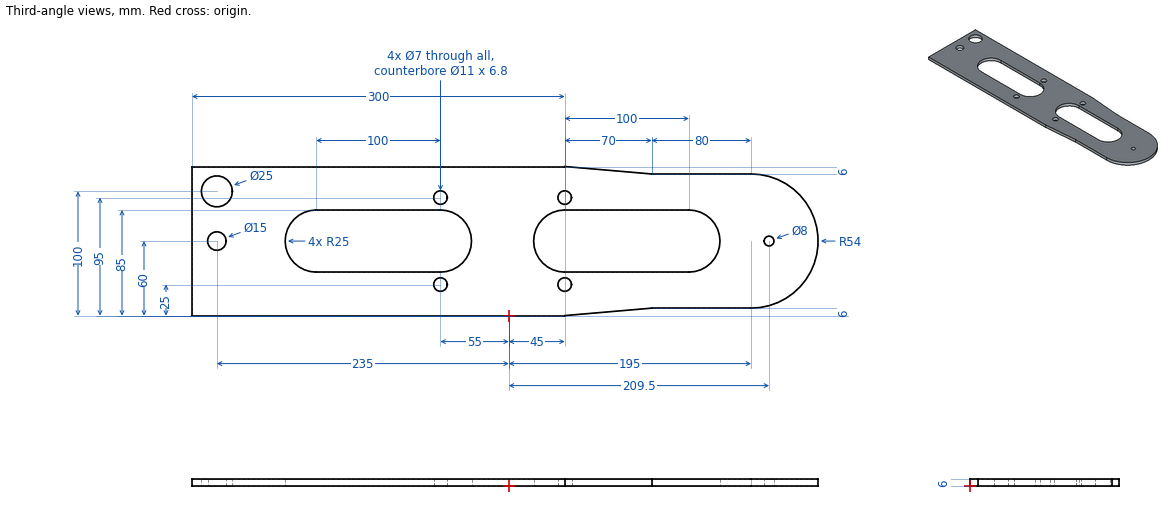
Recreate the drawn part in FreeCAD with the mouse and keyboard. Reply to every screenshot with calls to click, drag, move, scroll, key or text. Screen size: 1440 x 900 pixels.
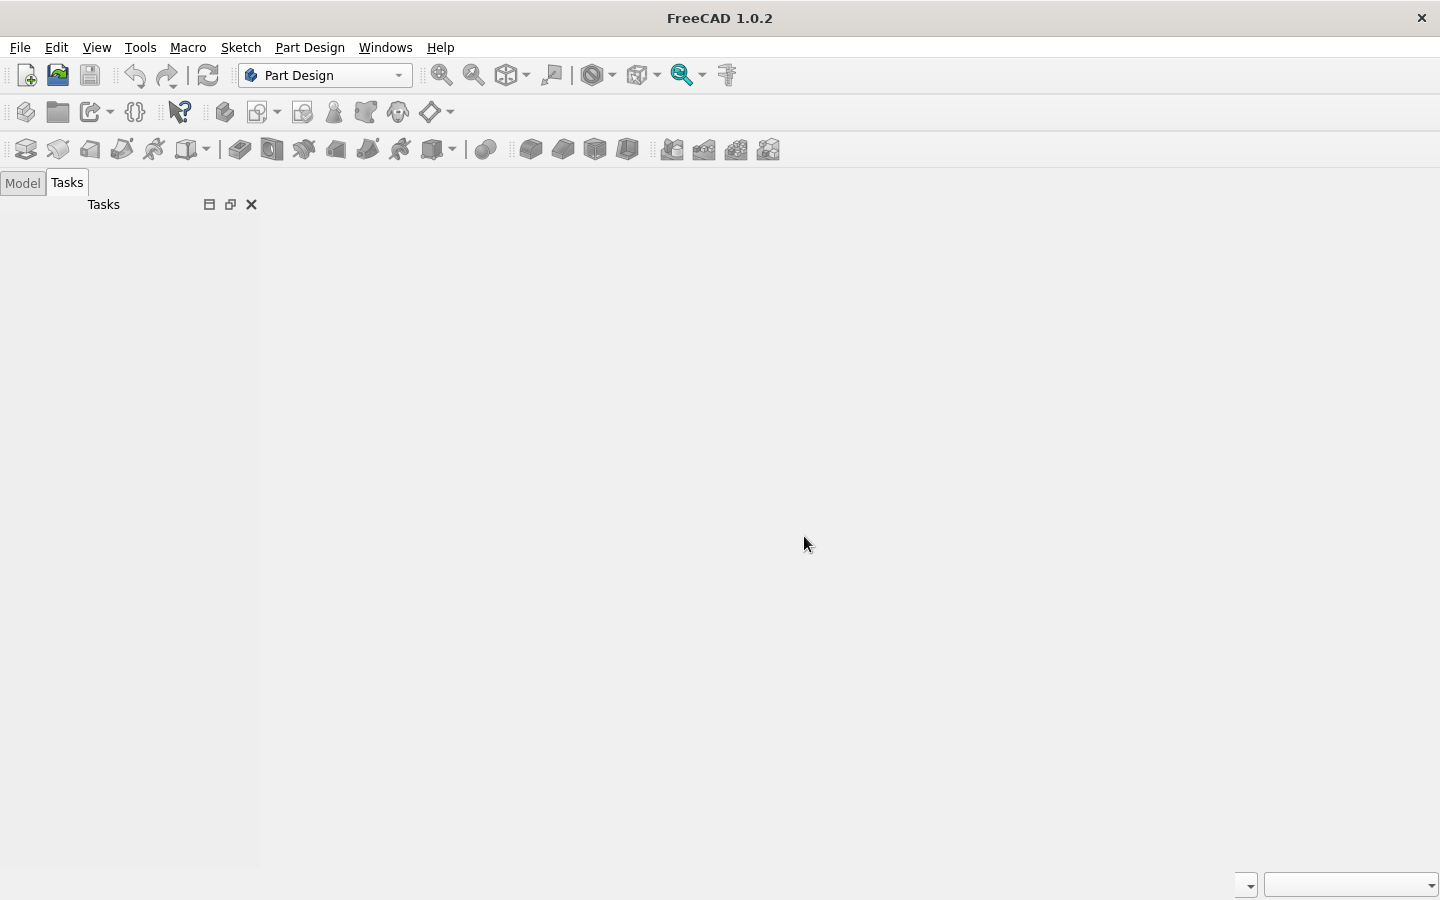
key(ctrl+n)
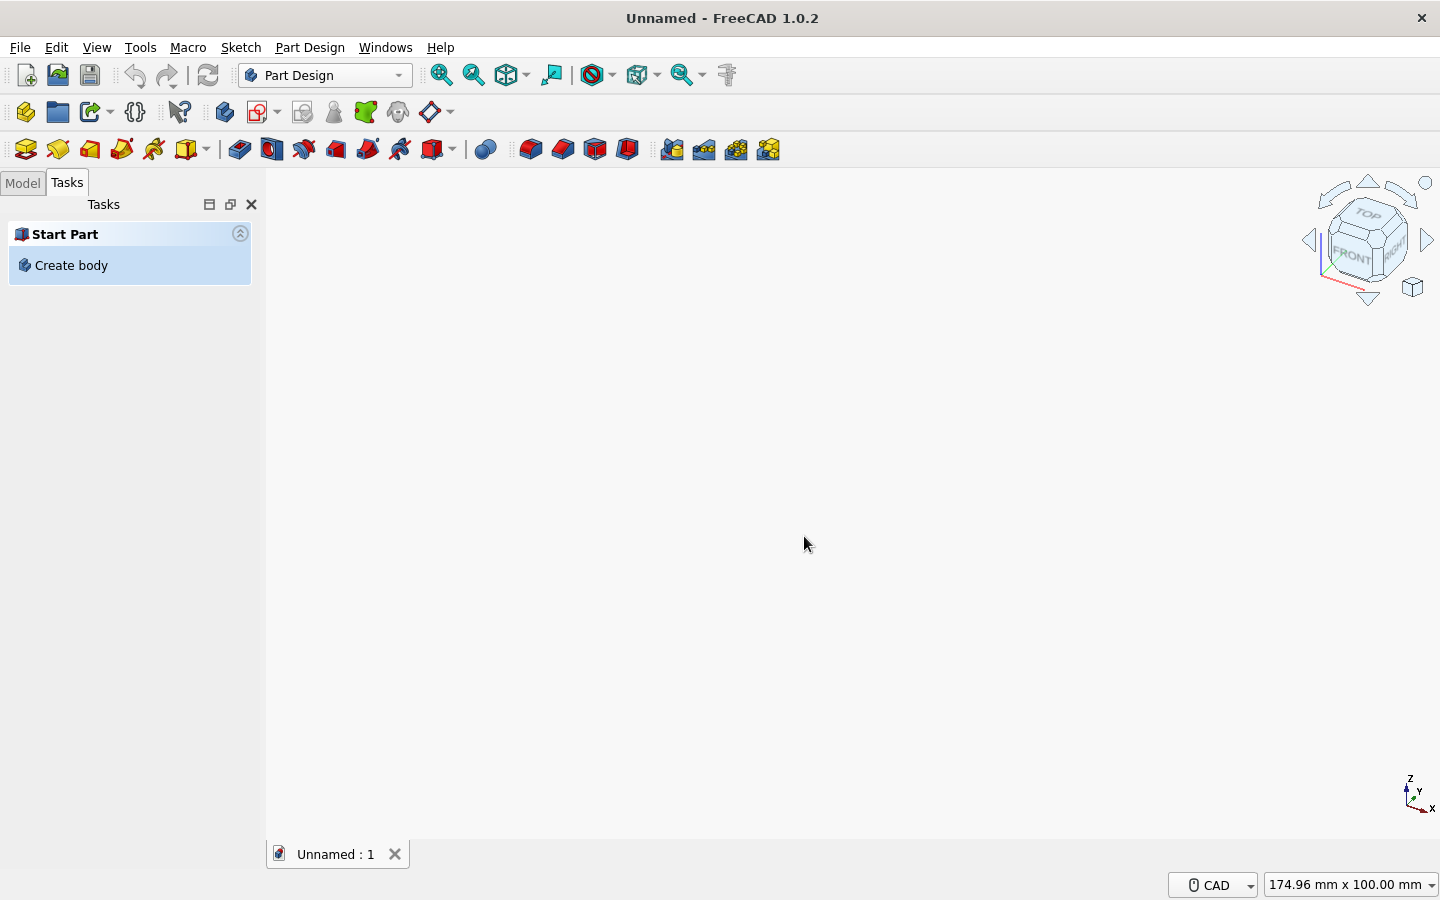
click(258, 112)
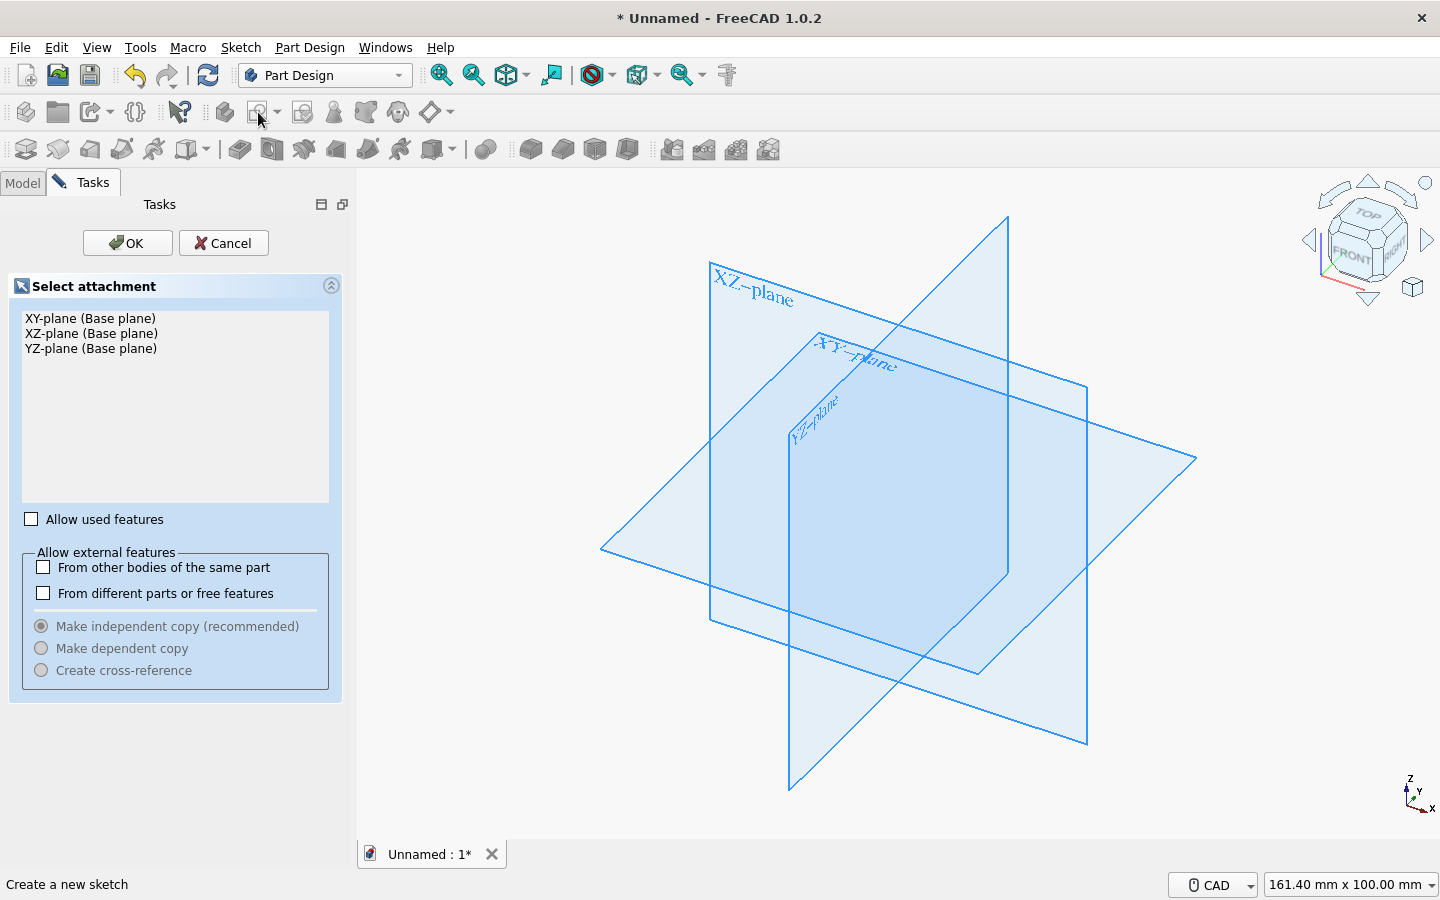
click(82, 318)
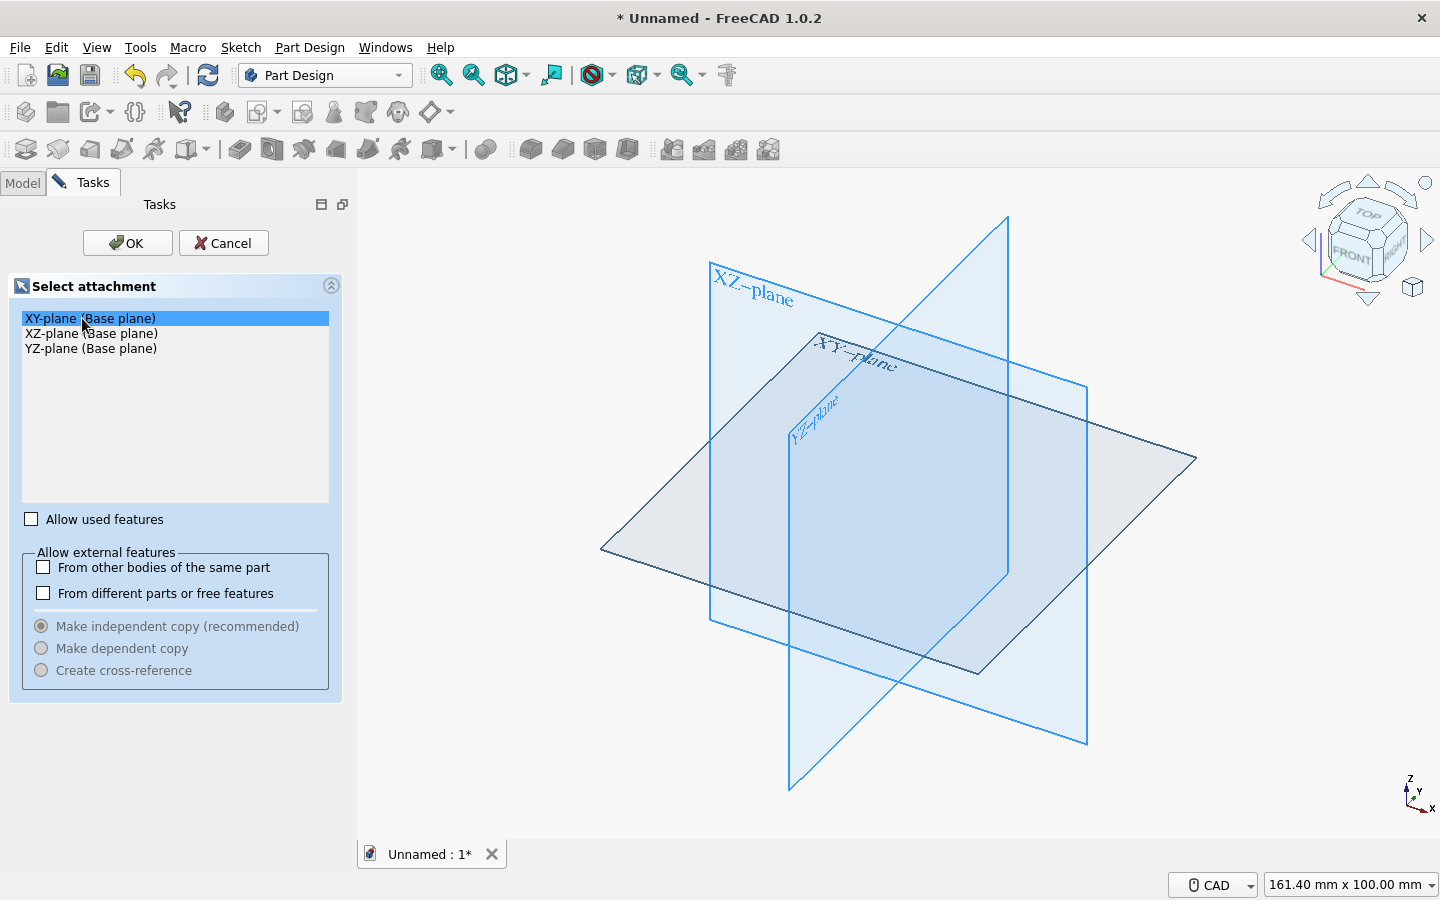
click(128, 243)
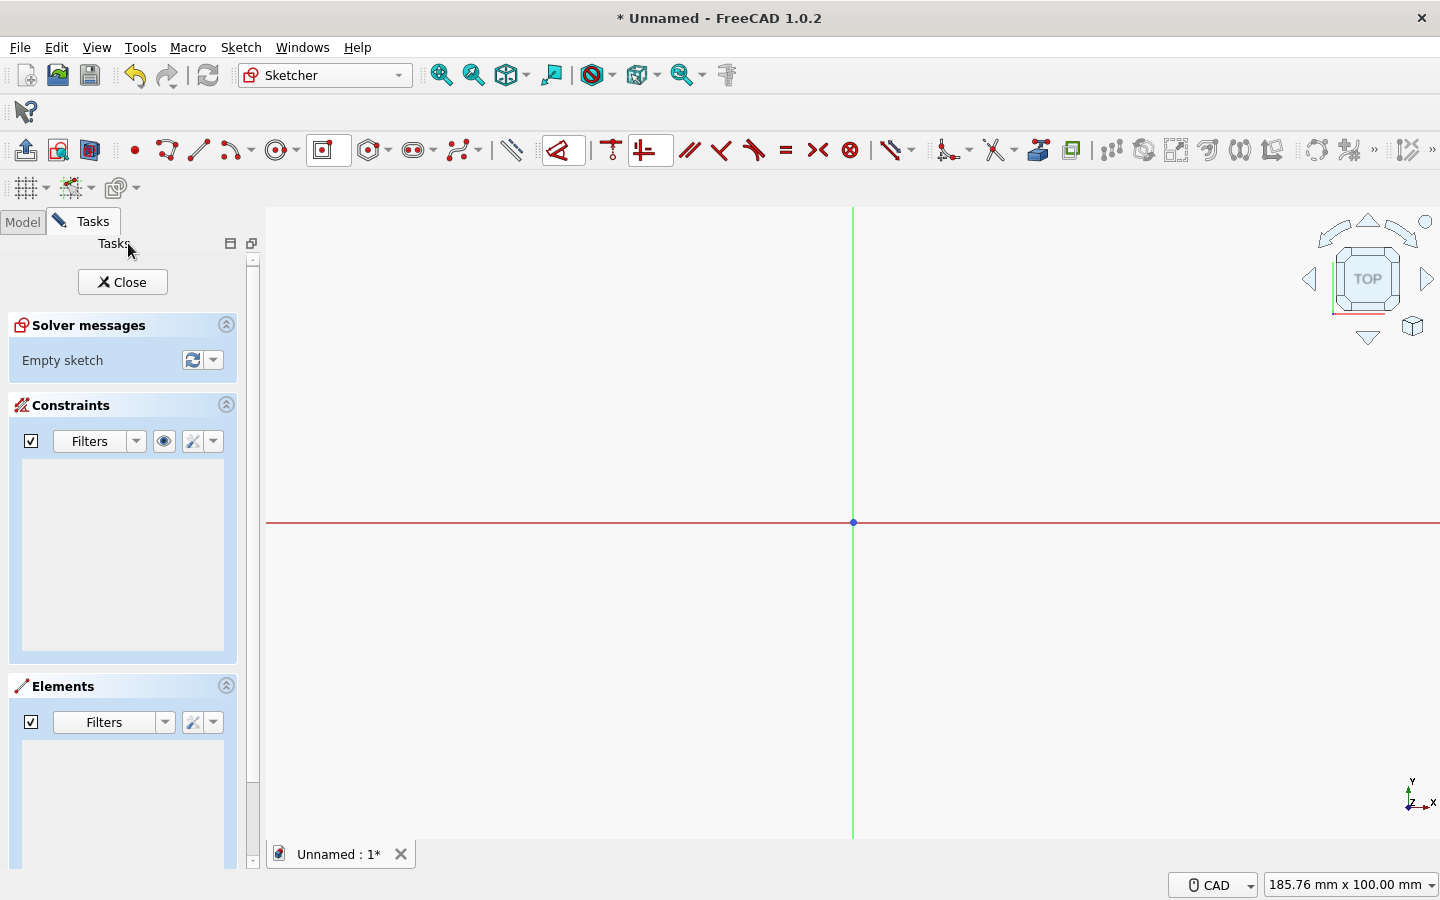
scroll(772, 619, down, 8)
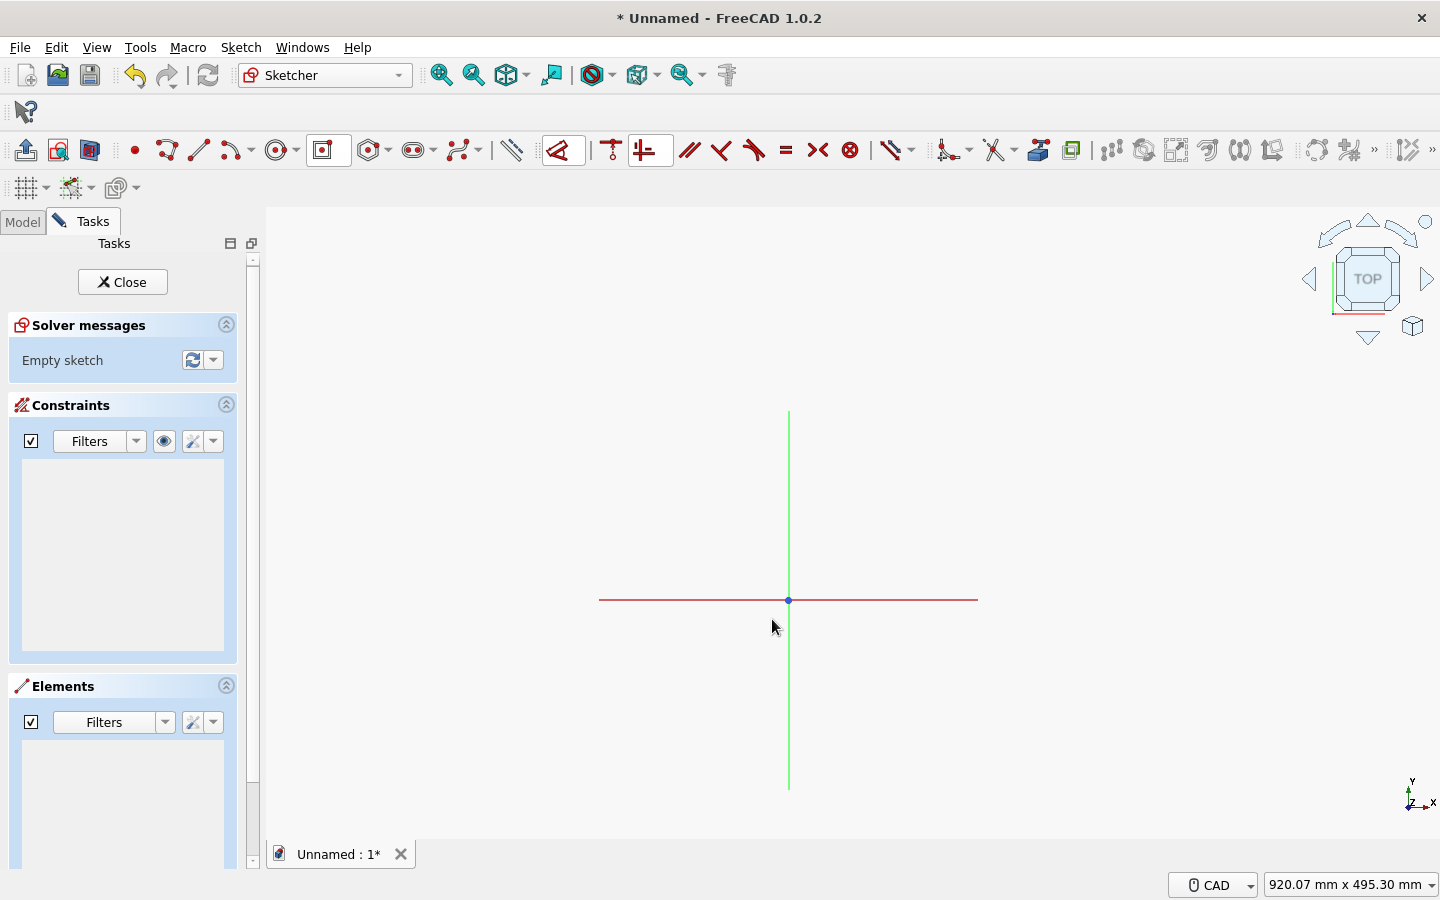
click(168, 150)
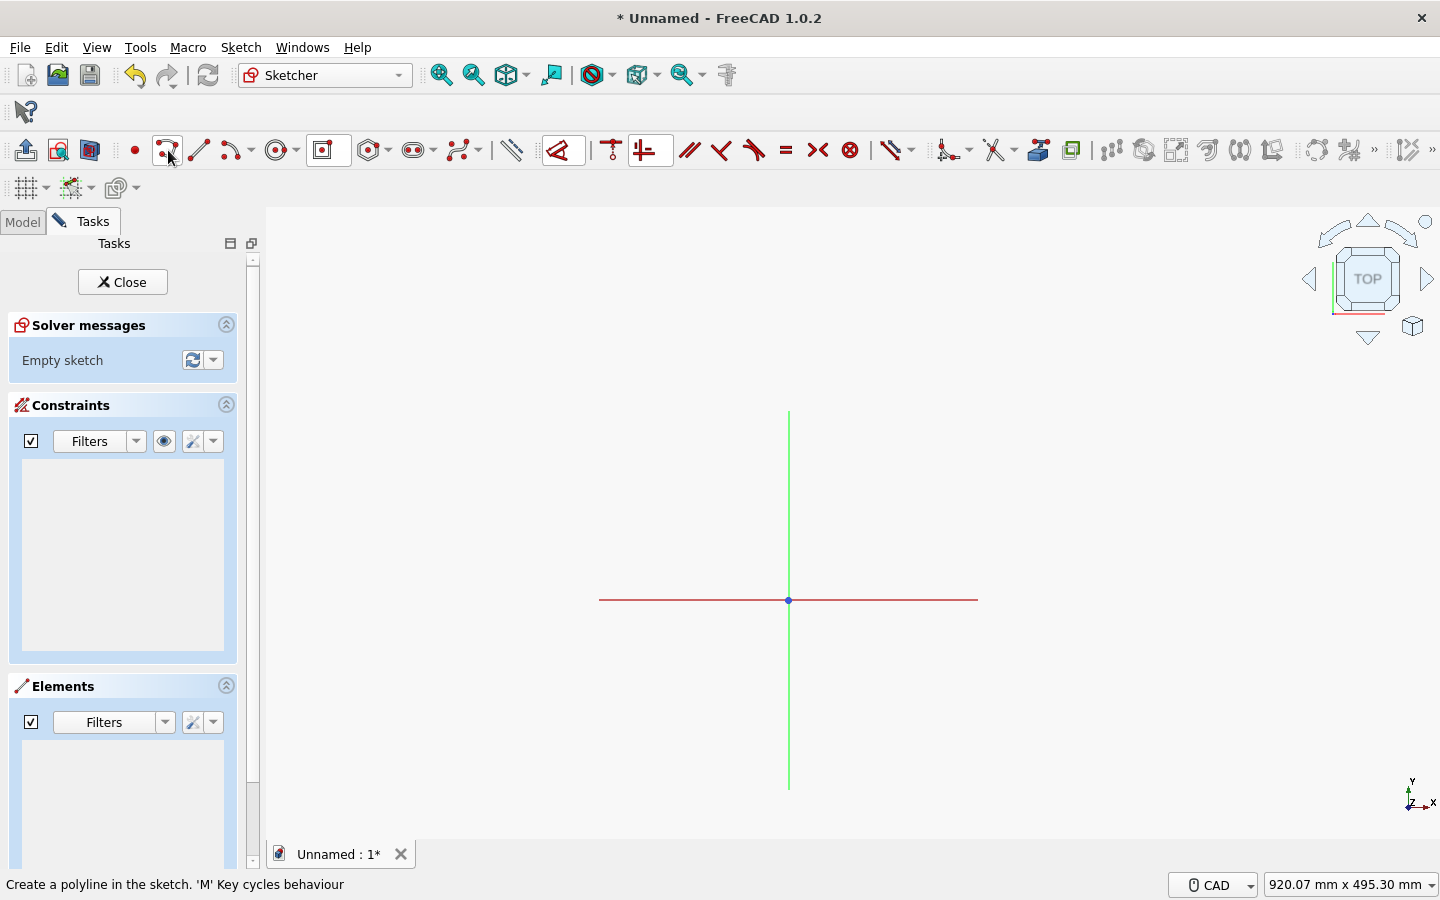
click(1038, 455)
click(935, 455)
click(846, 447)
click(463, 447)
click(463, 600)
click(846, 591)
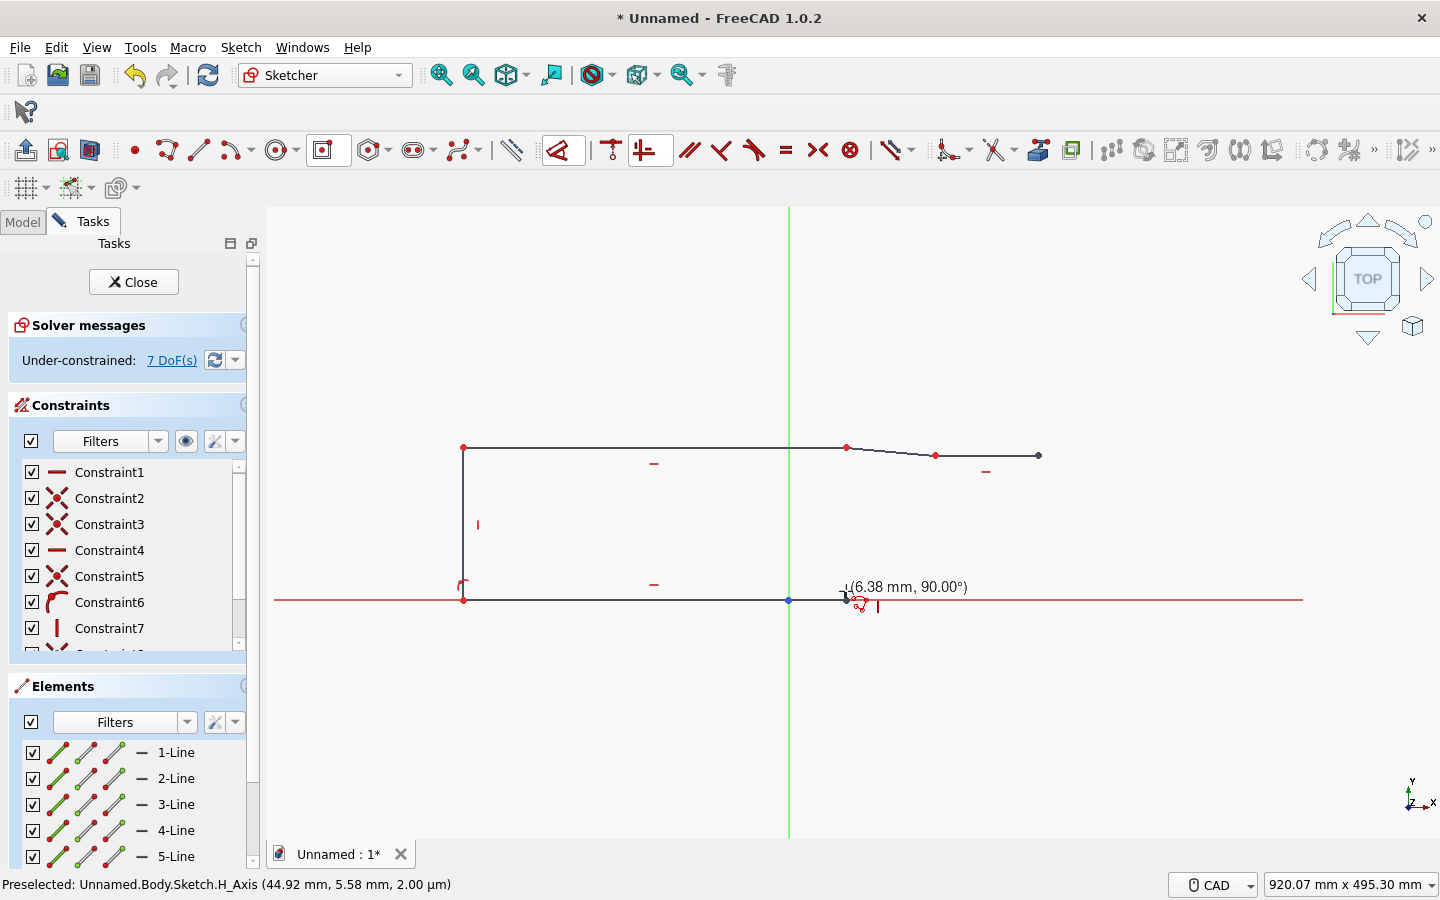
scroll(935, 592, up, 4)